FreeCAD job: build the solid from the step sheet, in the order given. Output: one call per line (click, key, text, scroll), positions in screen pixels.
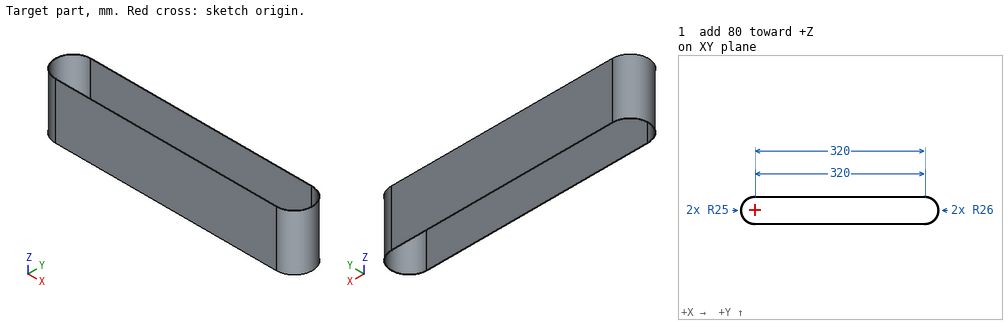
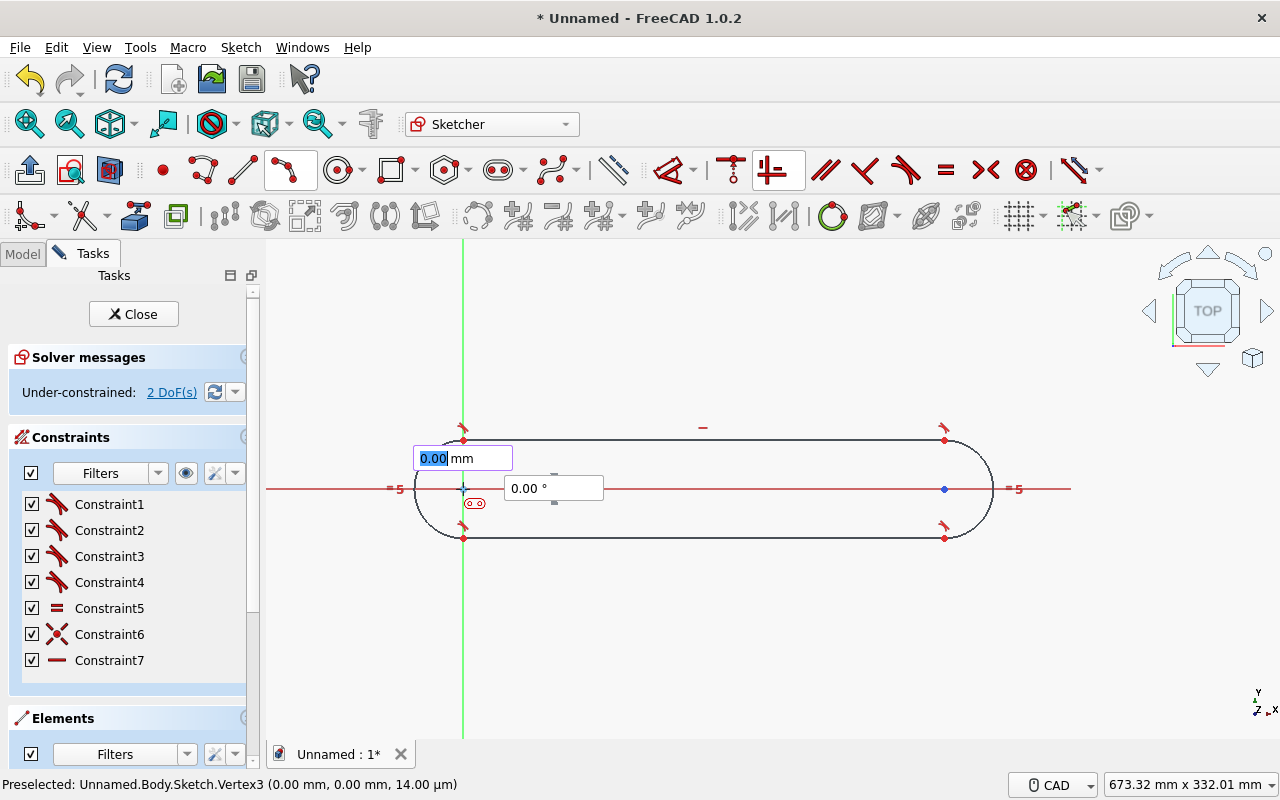
click(945, 480)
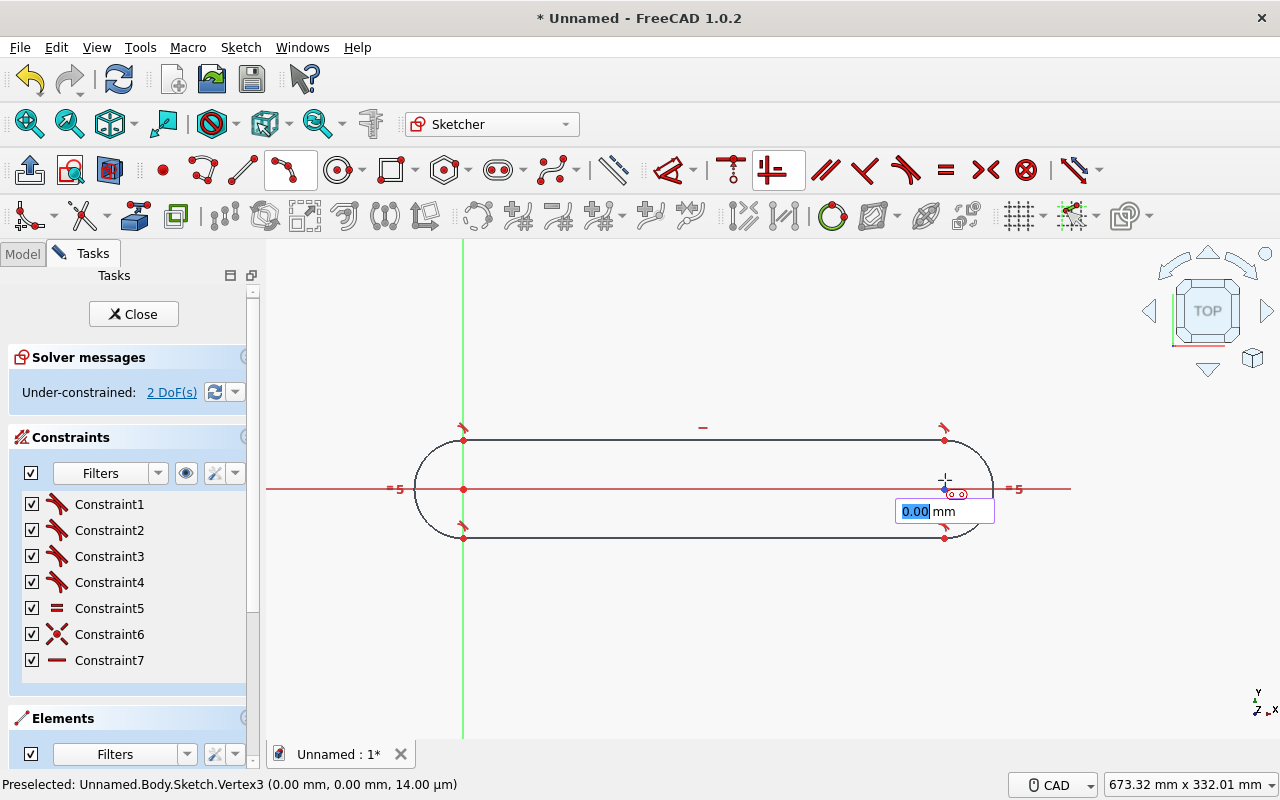
scroll(704, 452, up, 12)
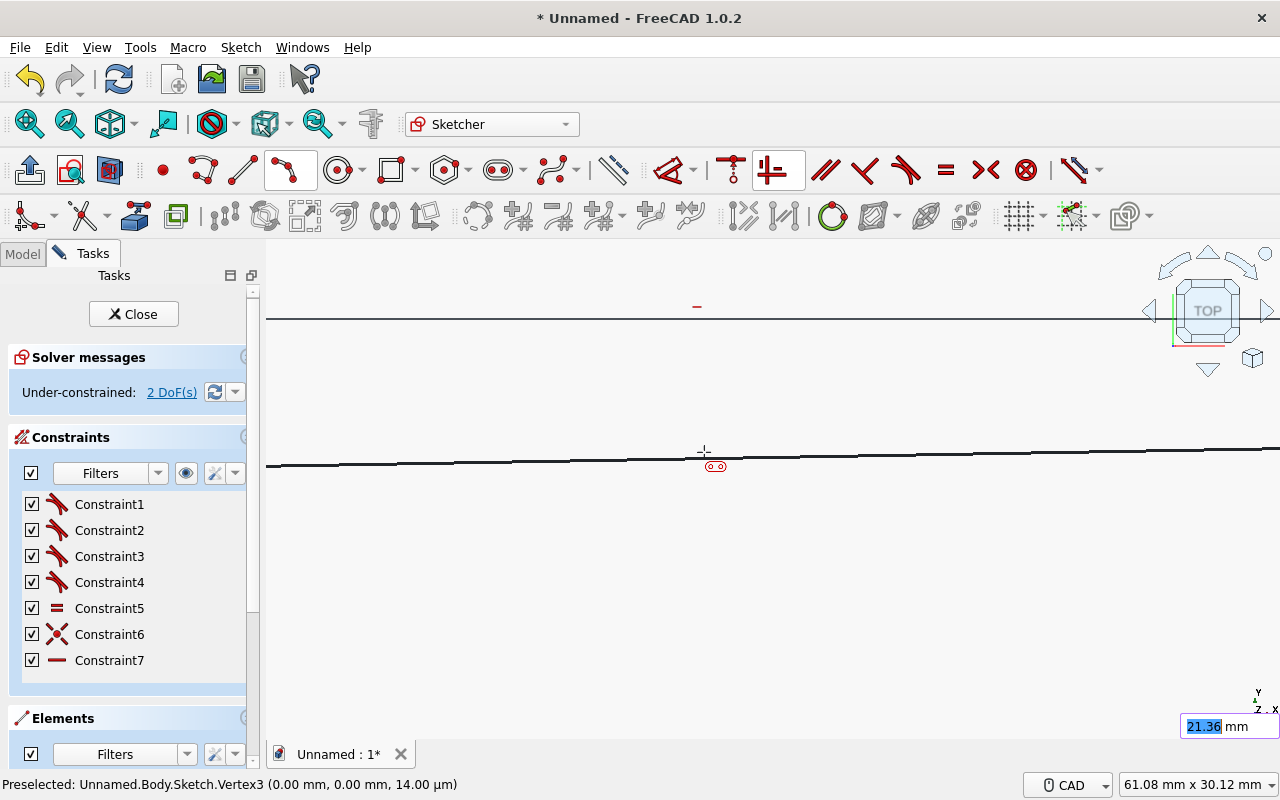
click(704, 444)
key(Escape)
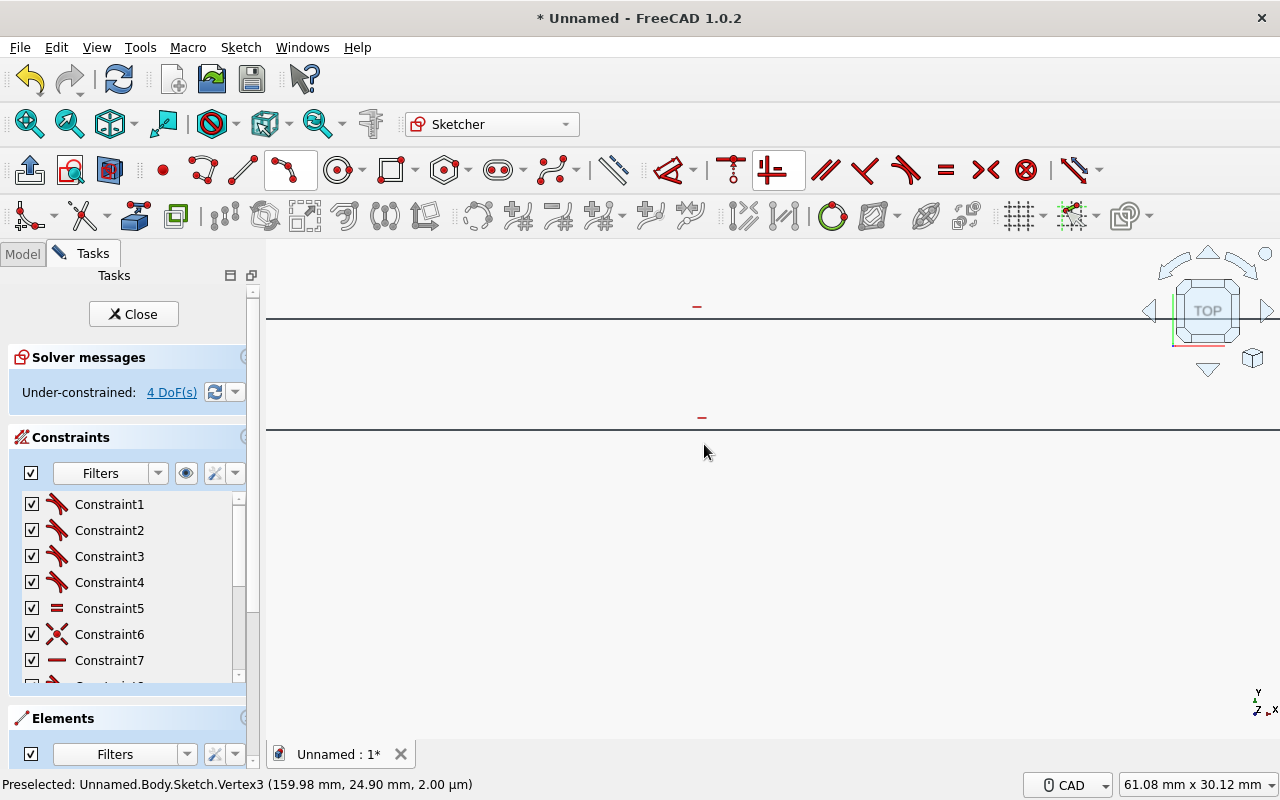
click(668, 170)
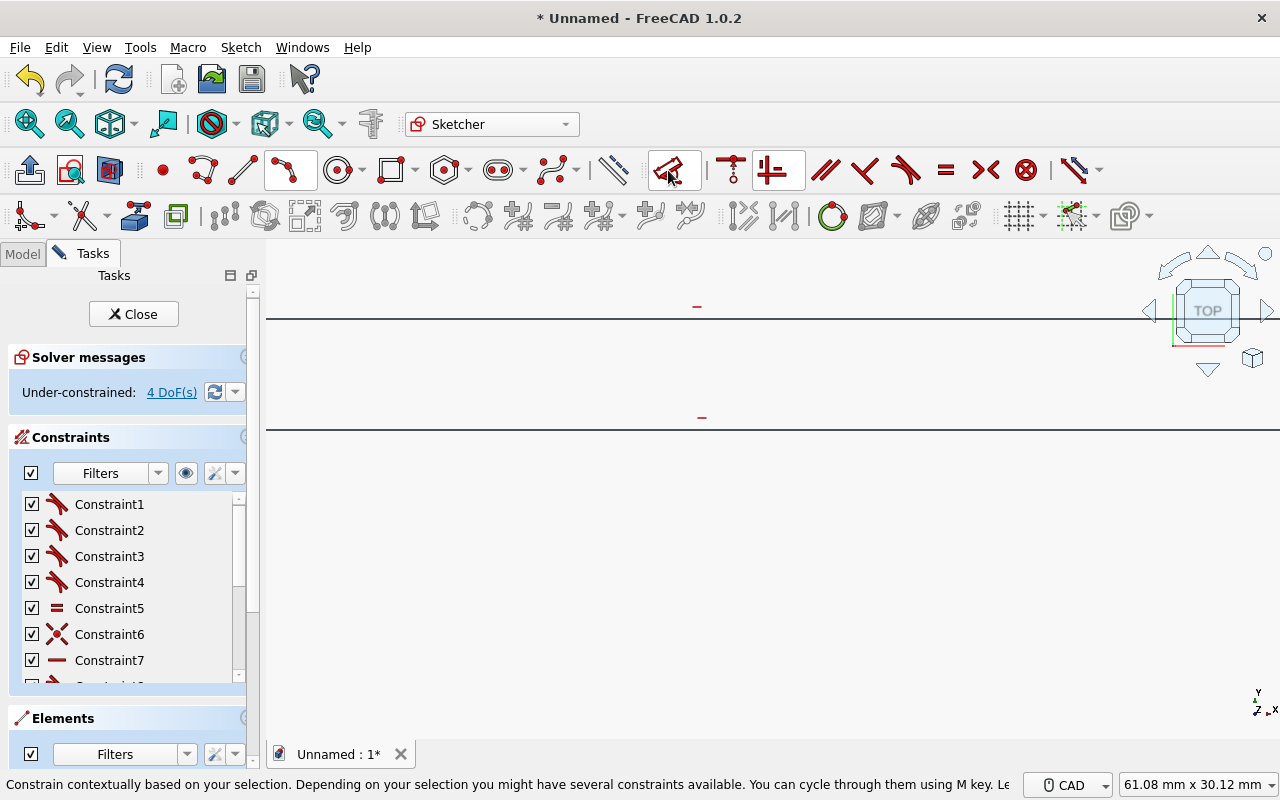
scroll(705, 452, down, 12)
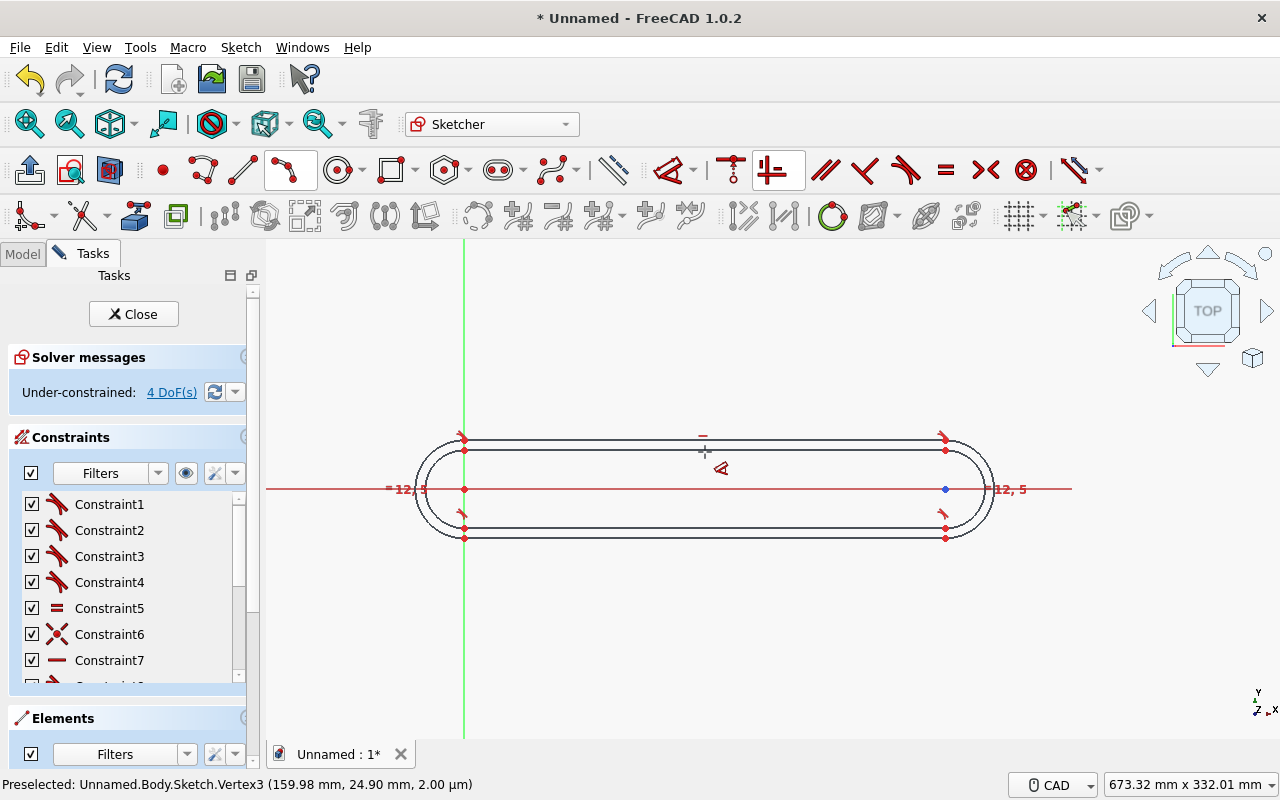
scroll(425, 461, up, 2)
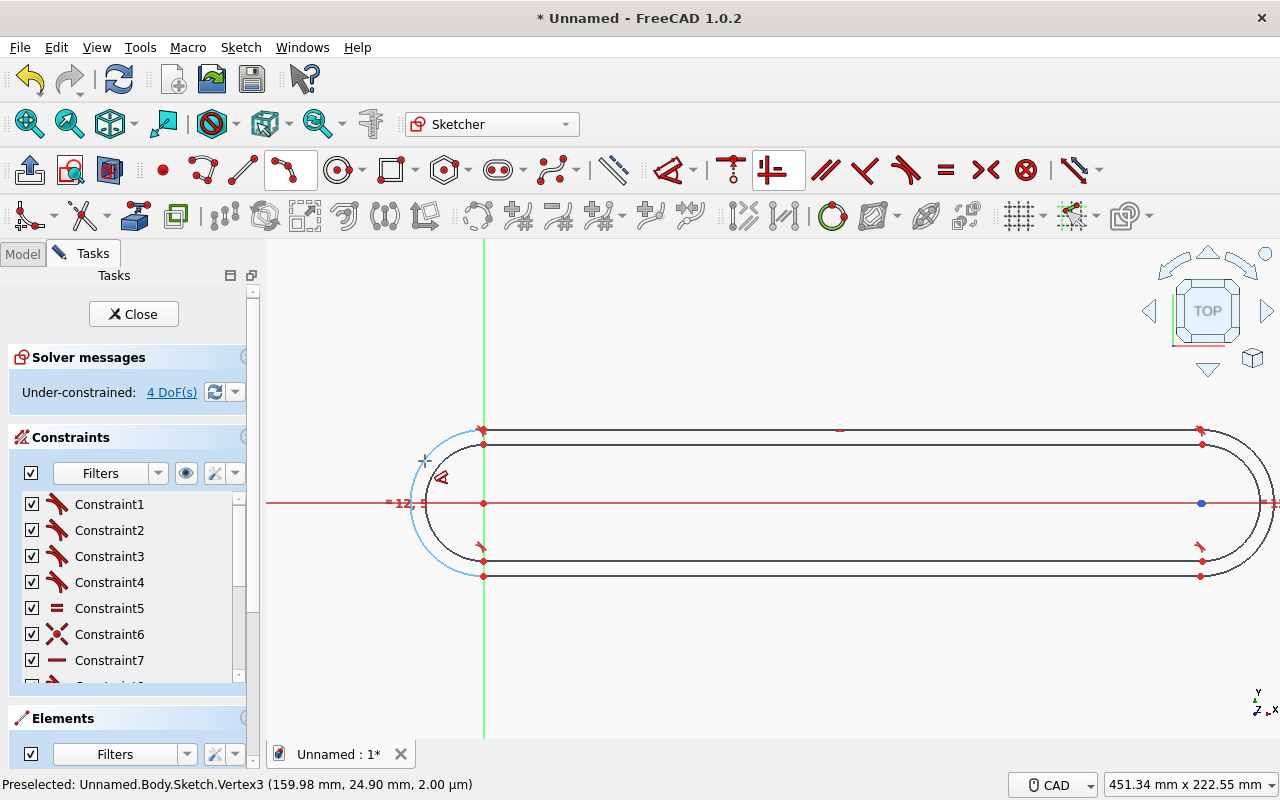
click(425, 460)
click(399, 441)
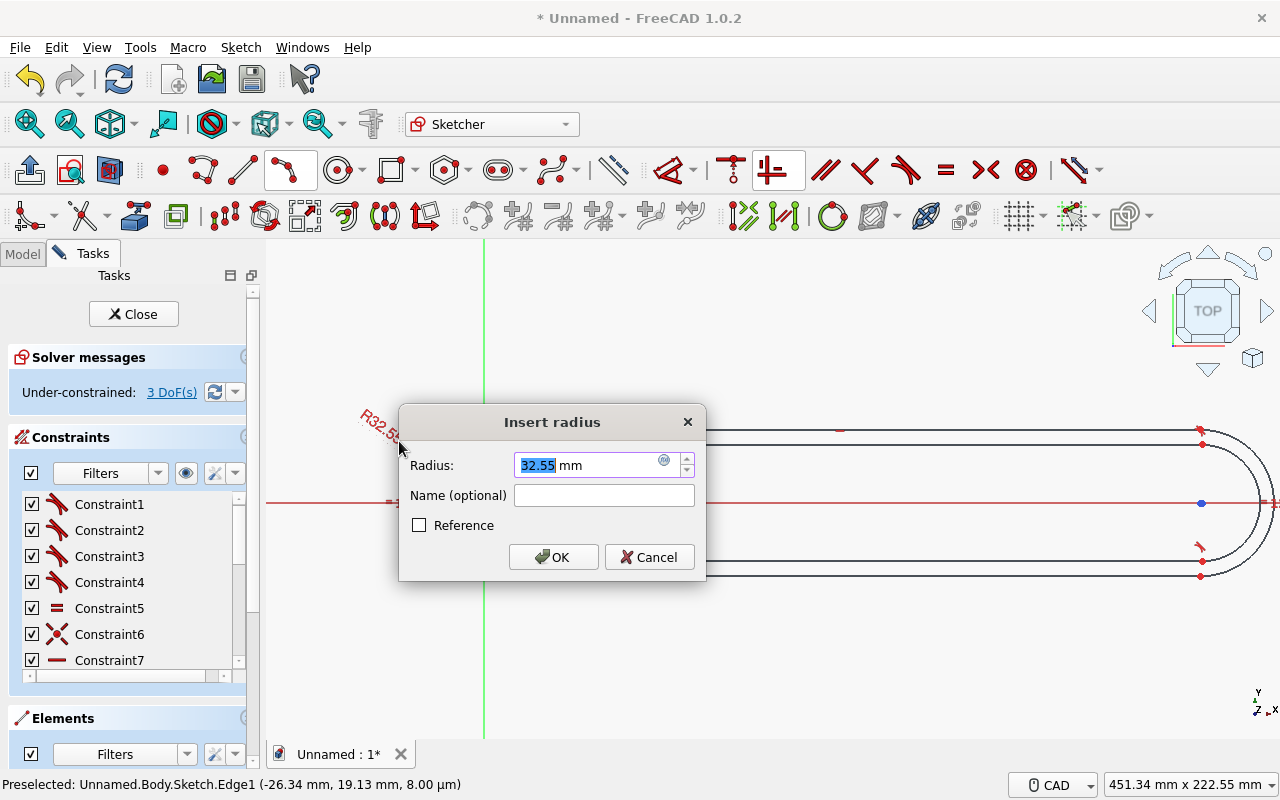
text(26)
key(Return)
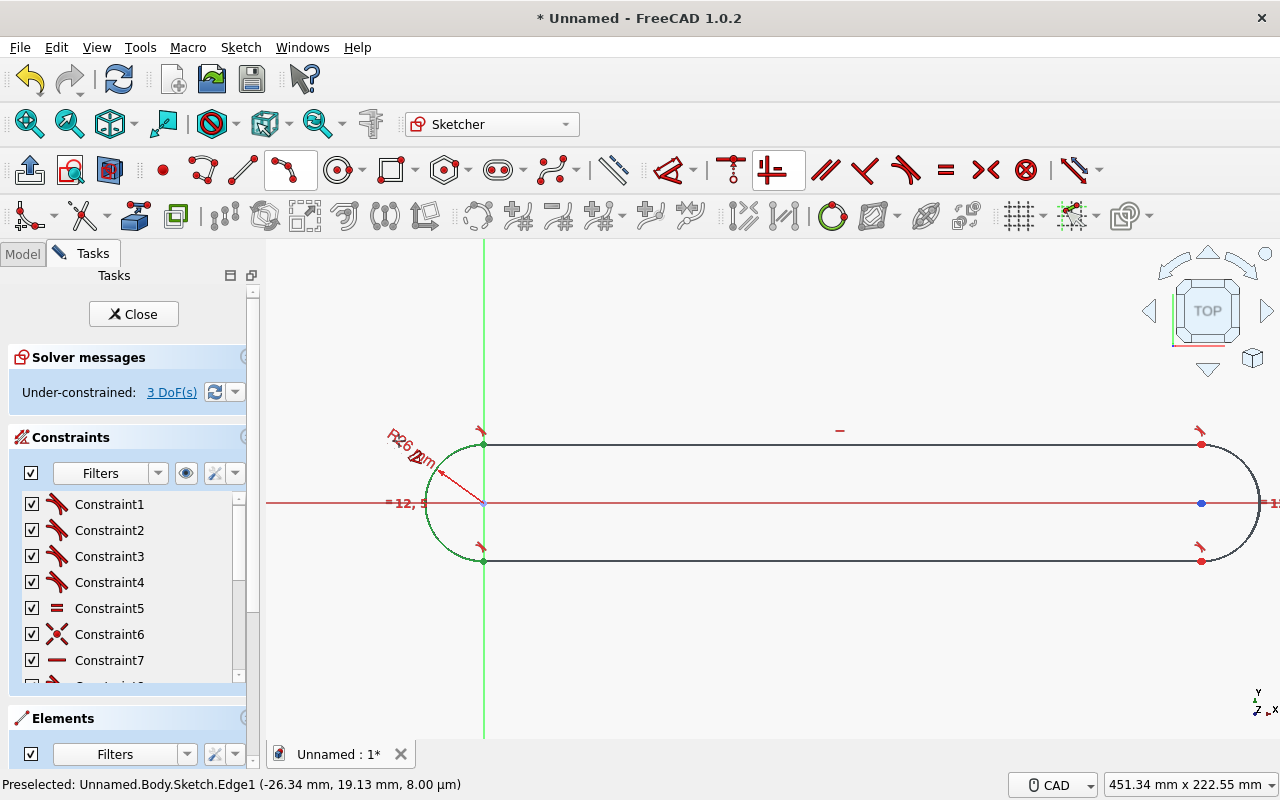
scroll(449, 456, up, 12)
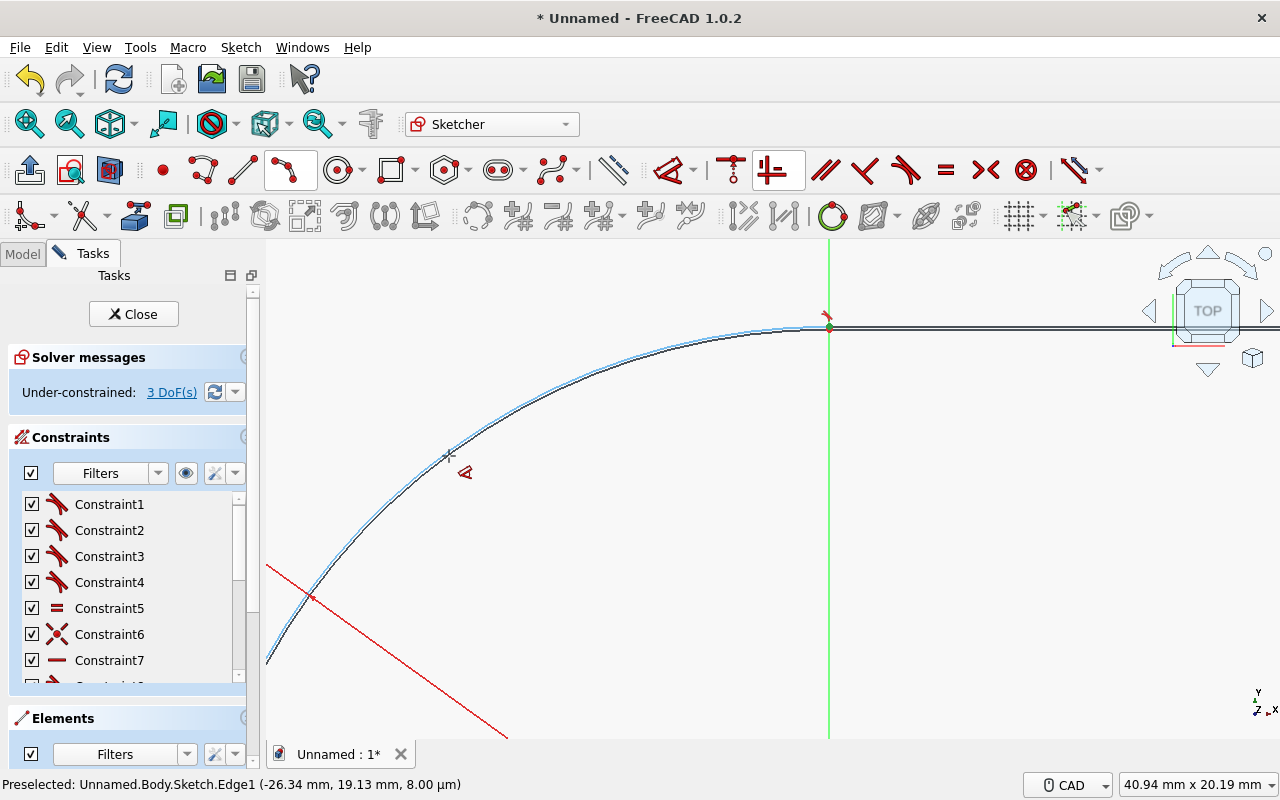
click(453, 452)
click(434, 426)